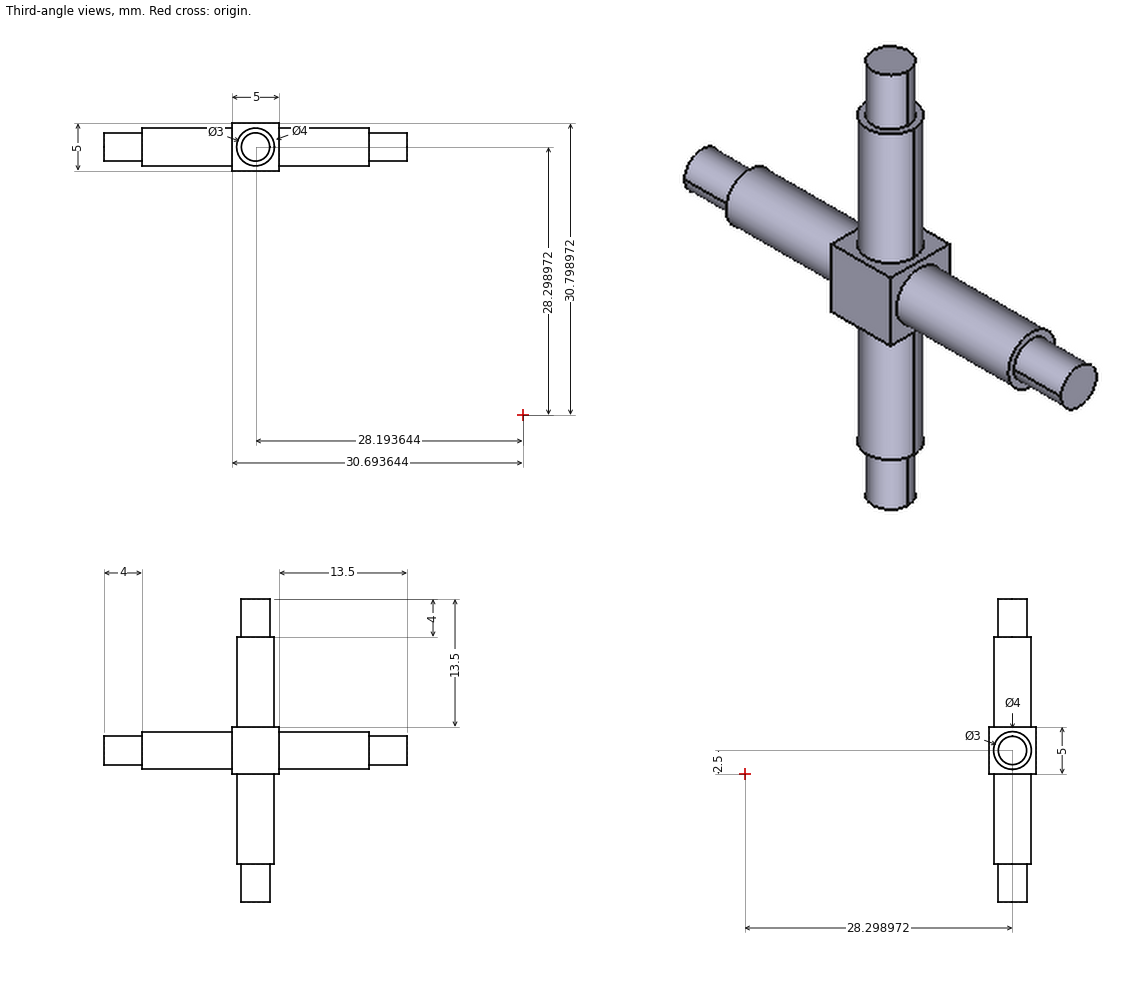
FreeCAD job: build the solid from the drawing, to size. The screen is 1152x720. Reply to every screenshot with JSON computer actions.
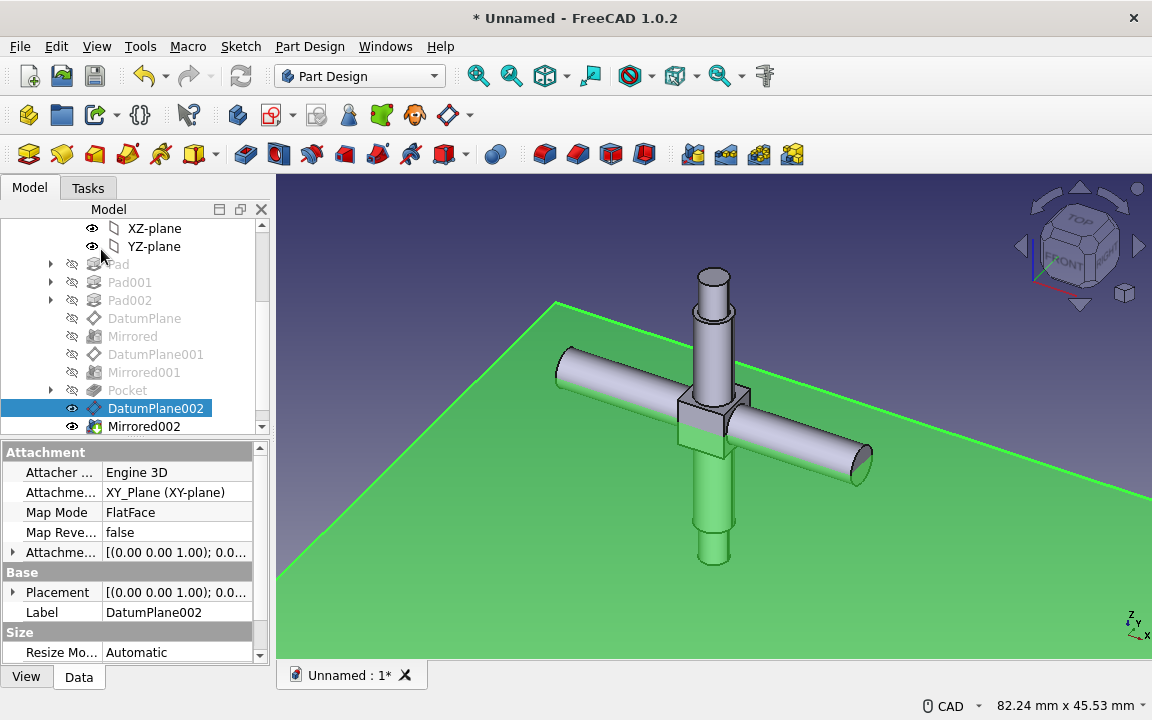
{"action": "left_click", "coordinate": [117, 408]}
{"action": "key", "text": "space"}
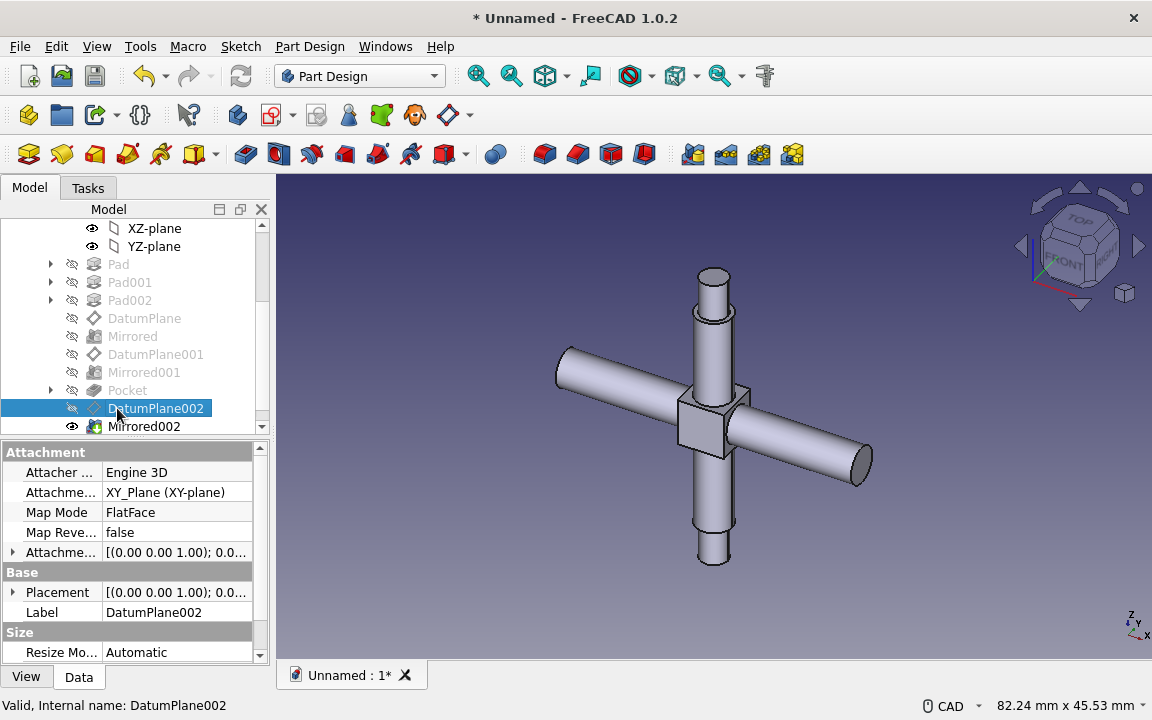
{"action": "key", "text": "6"}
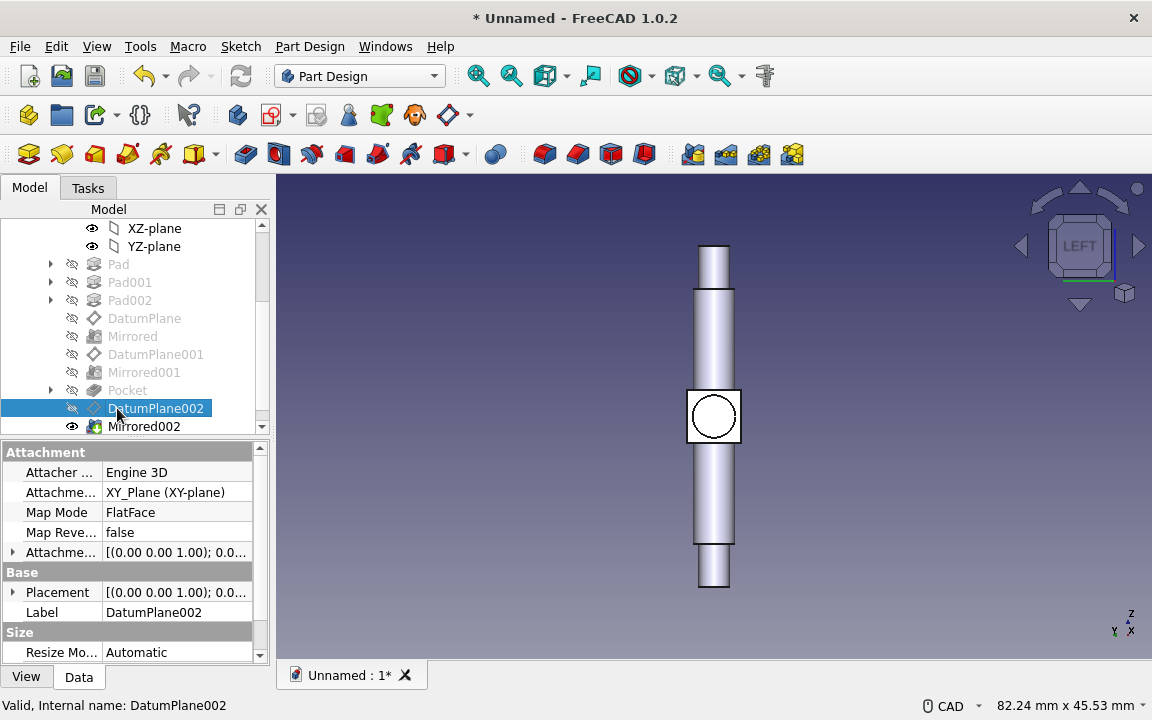
{"action": "left_click", "coordinate": [714, 415]}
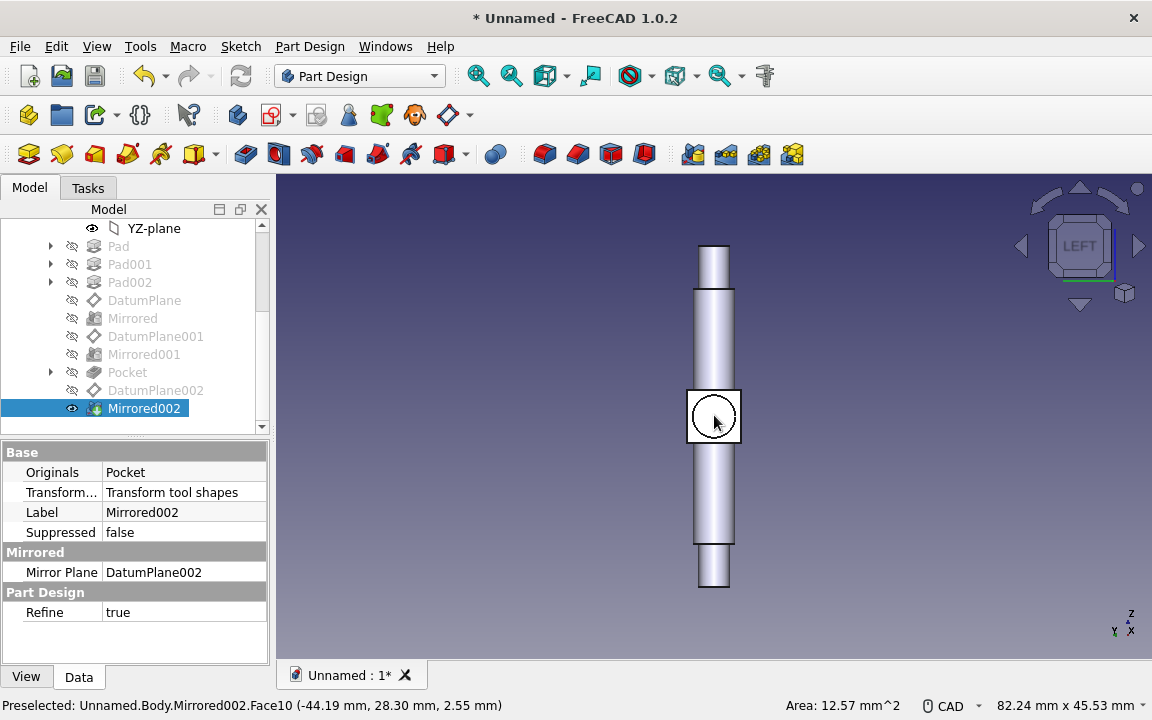
{"action": "left_click", "coordinate": [270, 116]}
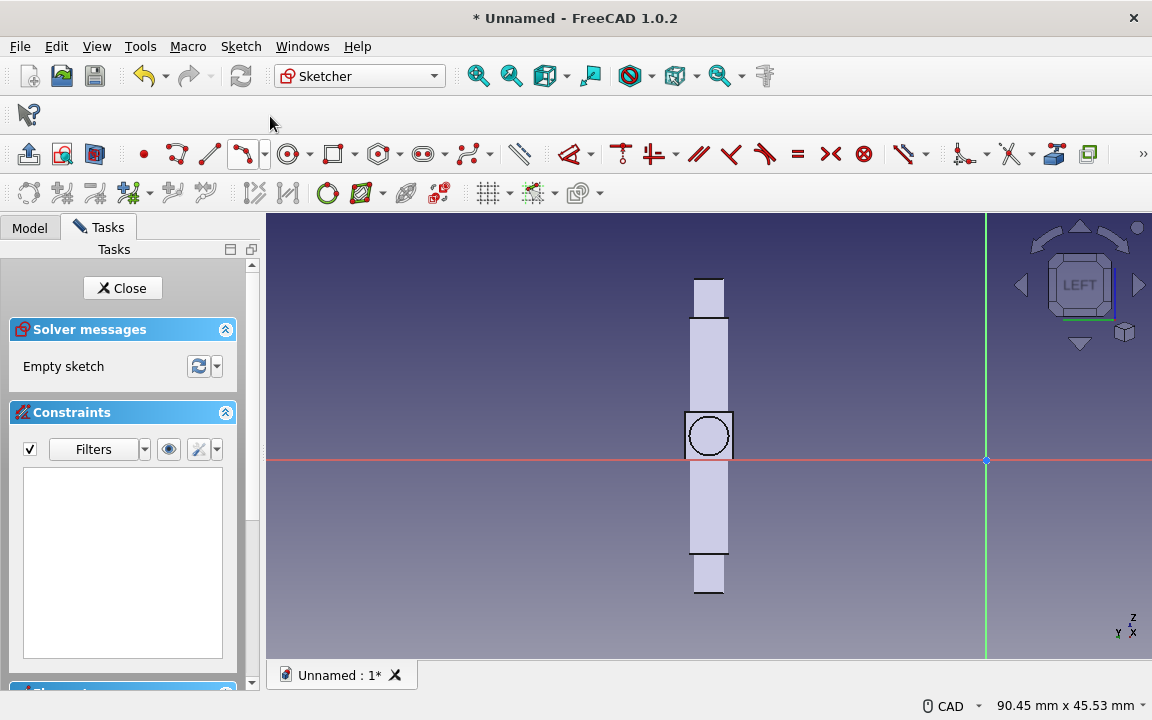
{"action": "scroll", "coordinate": [720, 436], "scroll_direction": "up", "scroll_amount": 10}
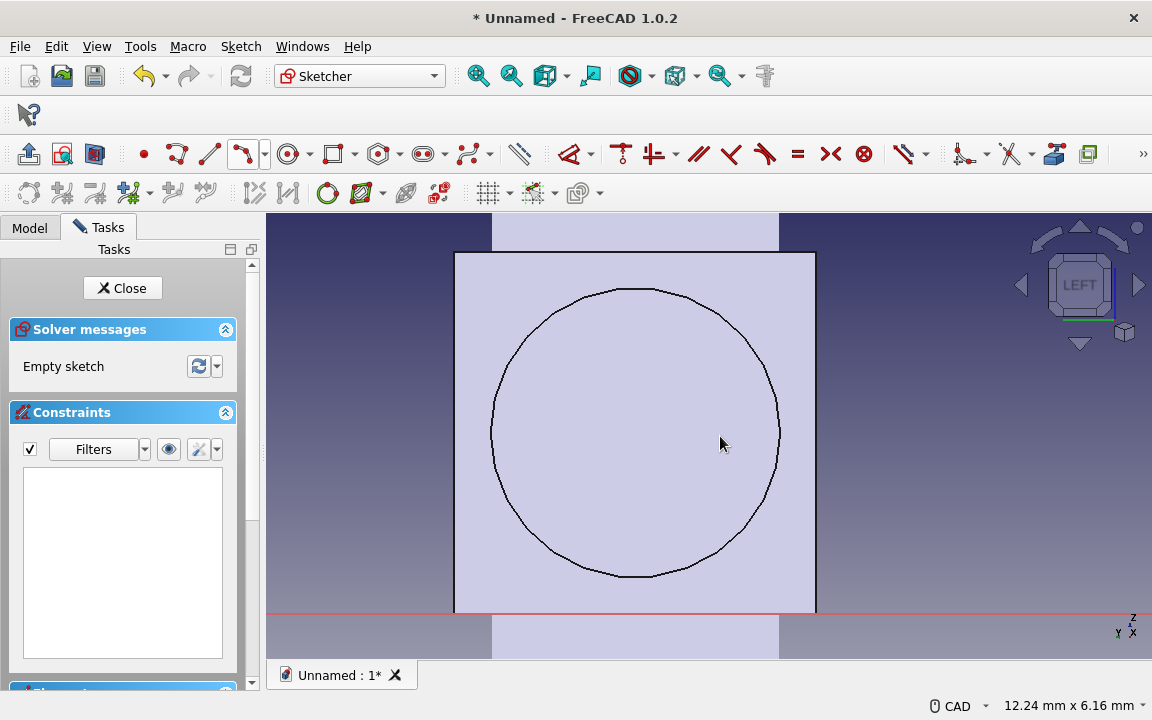
{"action": "left_click", "coordinate": [288, 154]}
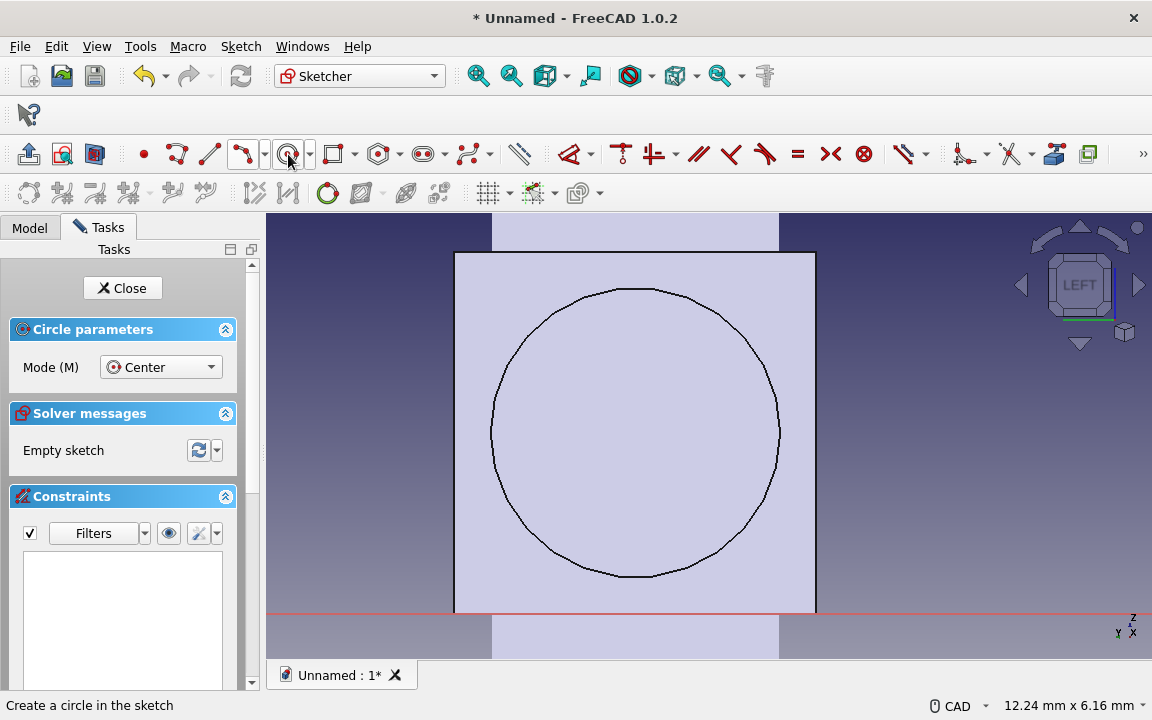
{"action": "left_click", "coordinate": [635, 433]}
{"action": "left_click", "coordinate": [738, 330]}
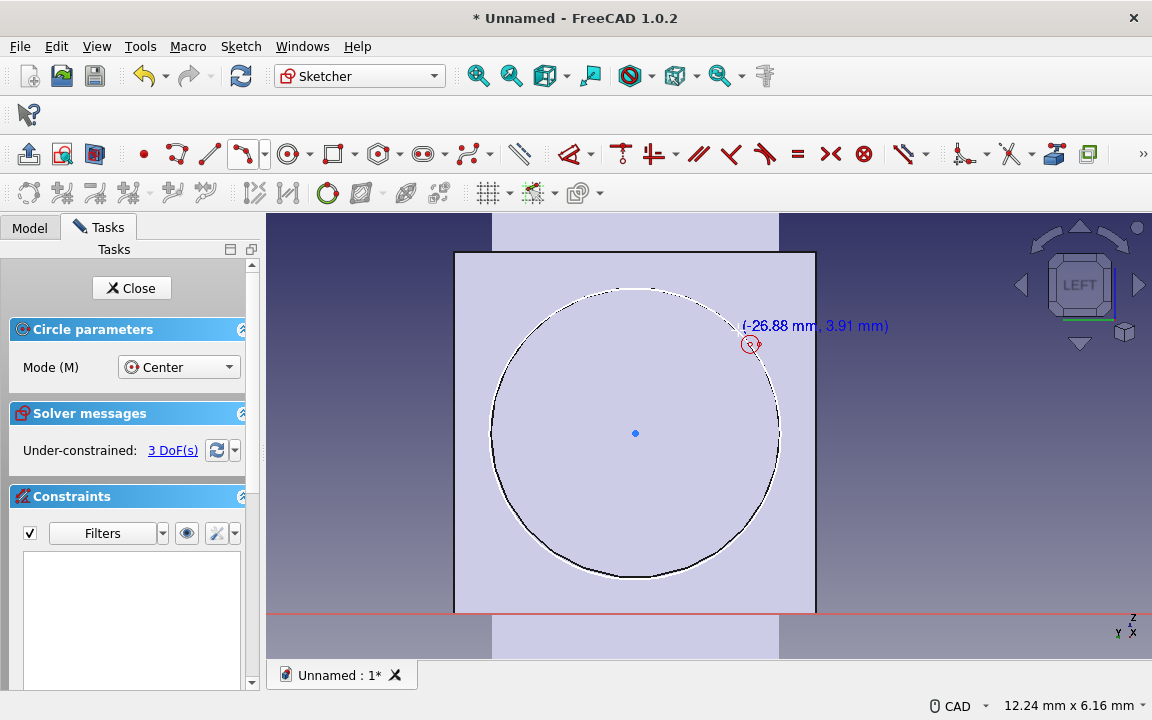
{"action": "left_click", "coordinate": [635, 434]}
{"action": "left_click", "coordinate": [712, 356]}
{"action": "key", "text": "Escape"}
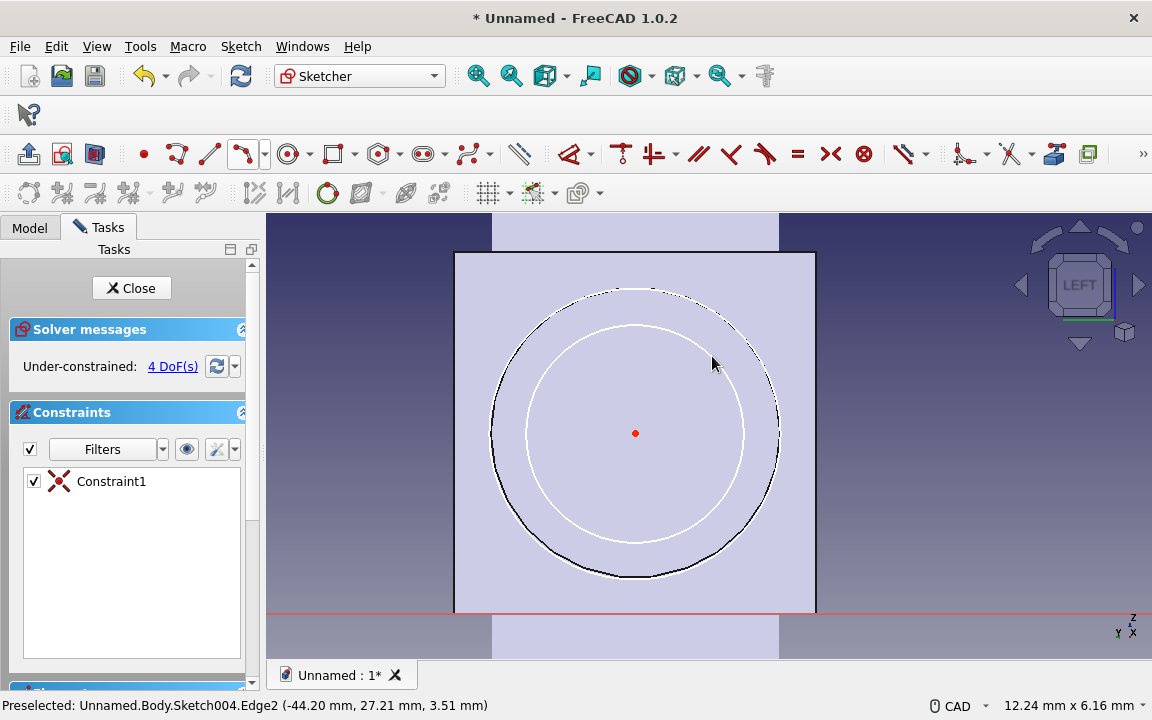
{"action": "key", "text": "d"}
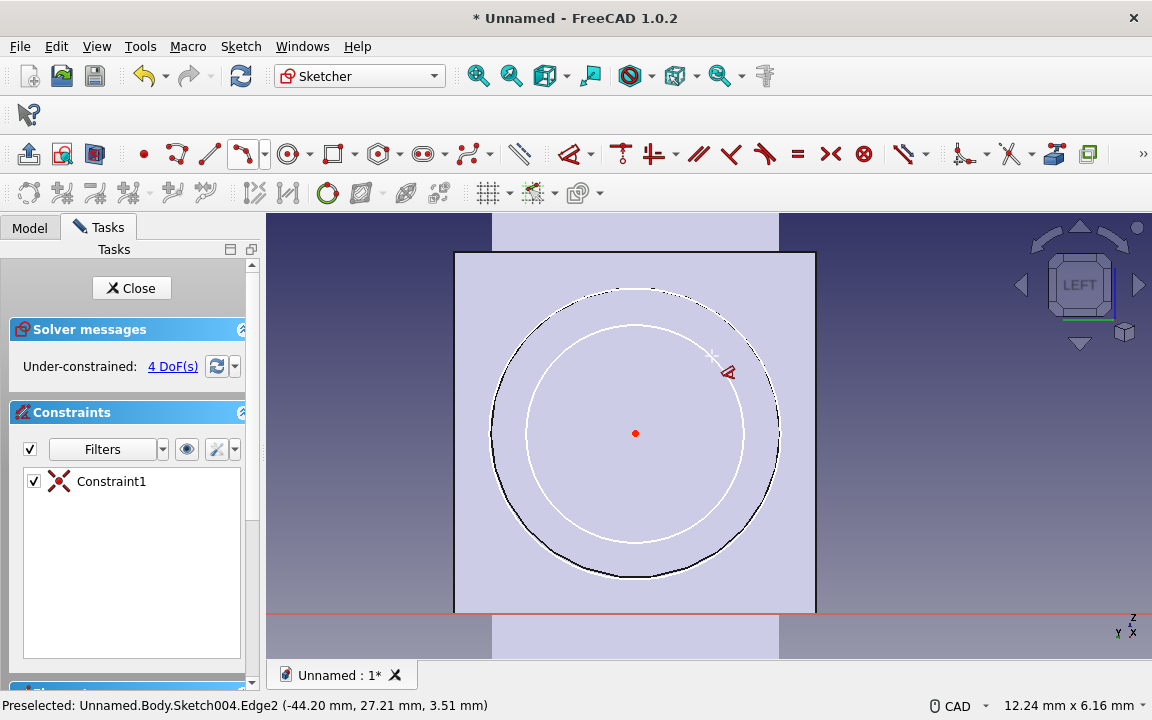
{"action": "left_click", "coordinate": [738, 331]}
{"action": "left_click", "coordinate": [761, 308]}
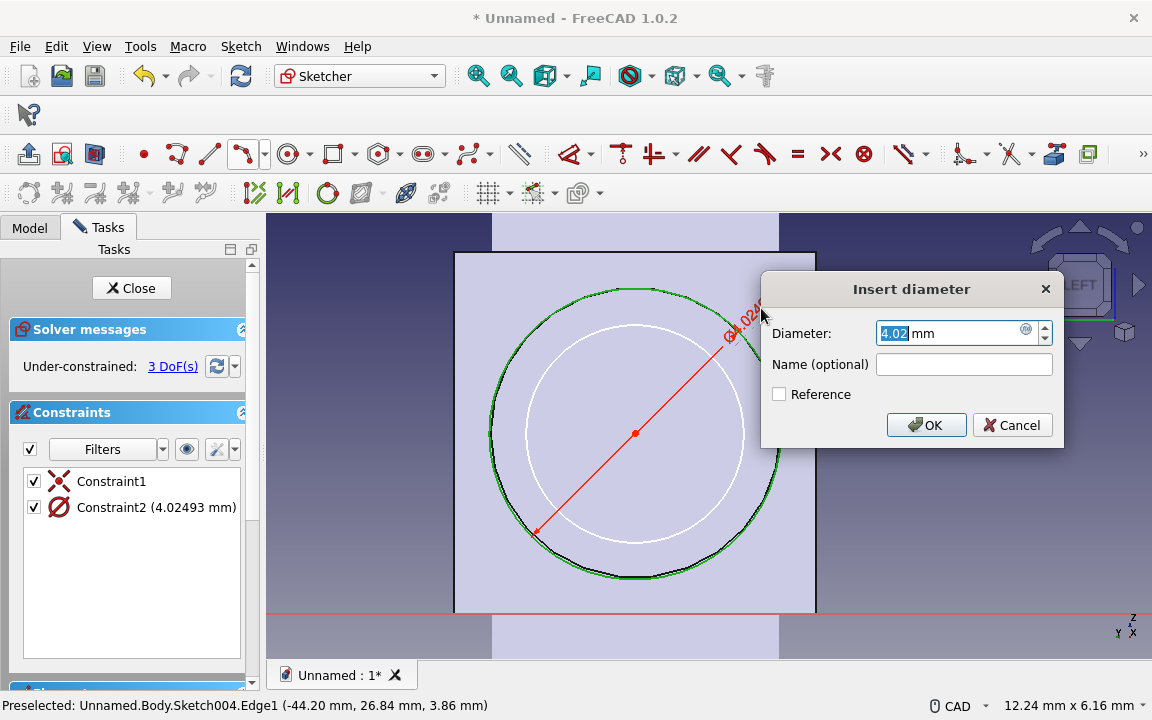
{"action": "type", "text": "4"}
{"action": "key", "text": "Return"}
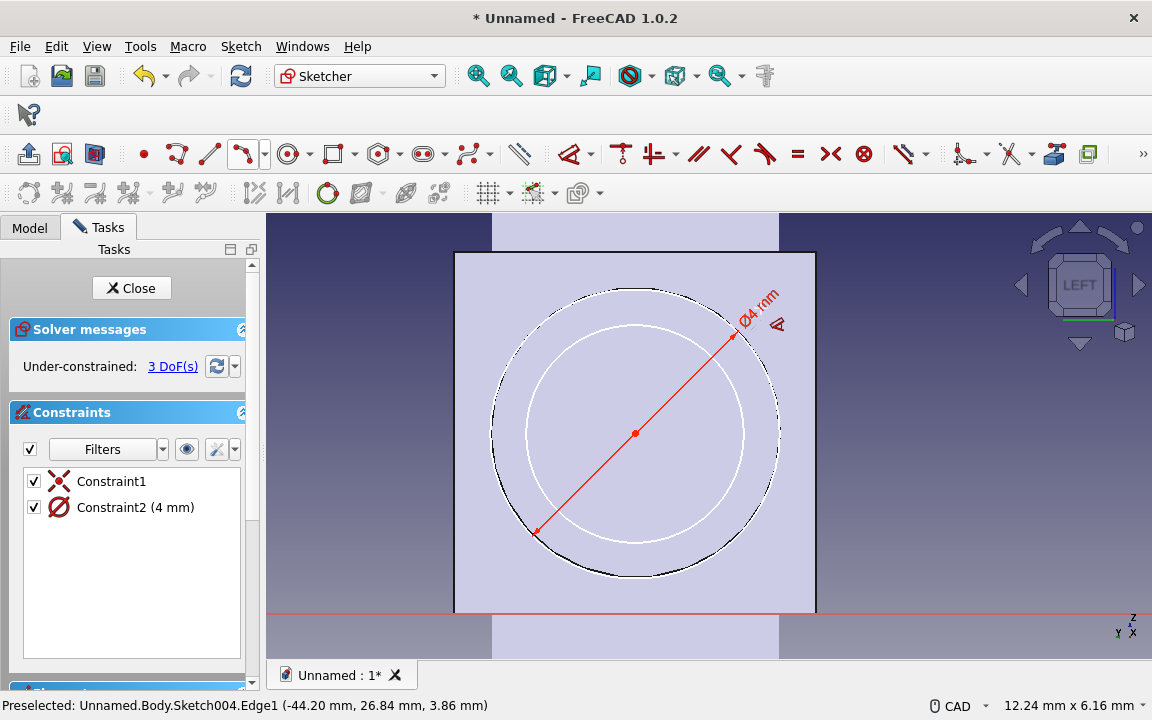
{"action": "left_click", "coordinate": [712, 357]}
{"action": "left_click", "coordinate": [792, 388]}